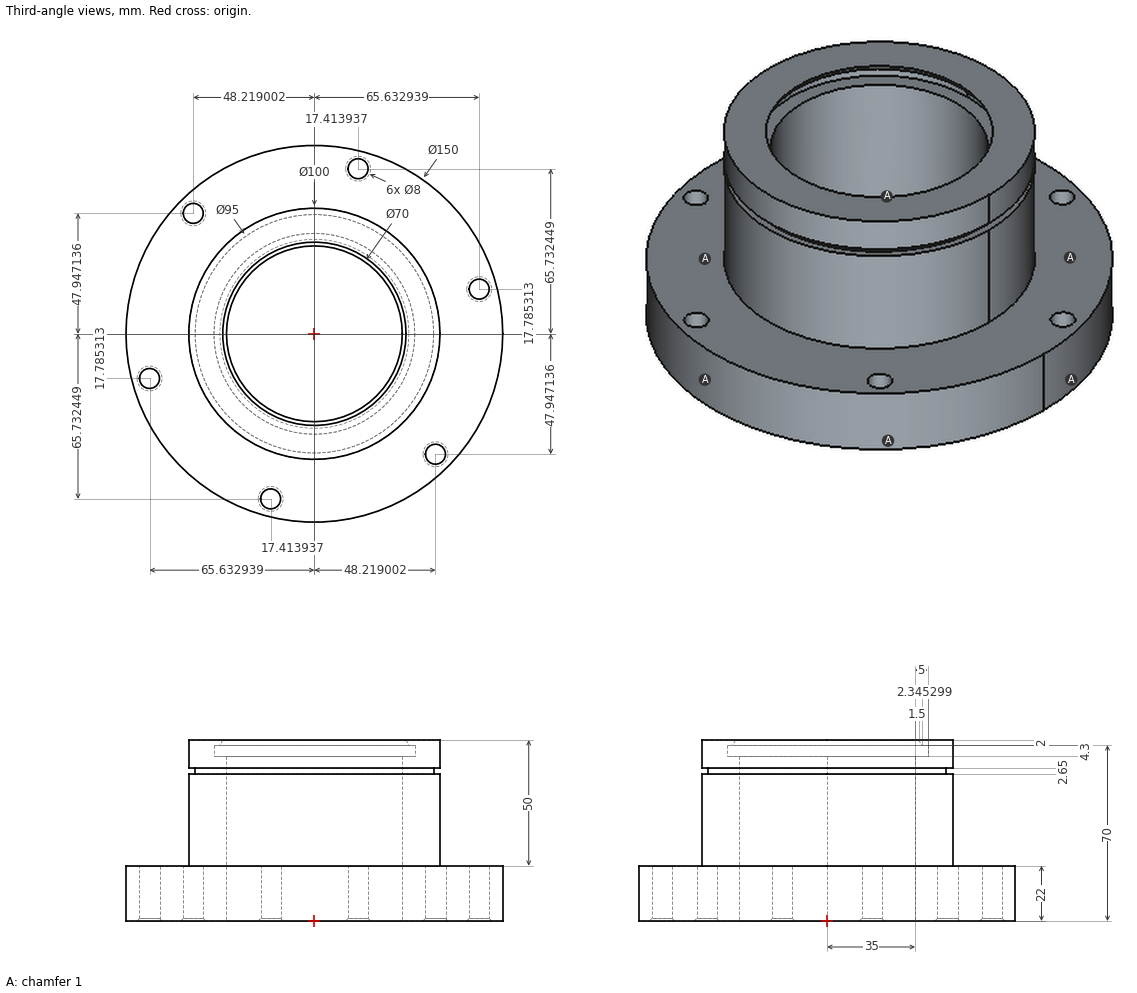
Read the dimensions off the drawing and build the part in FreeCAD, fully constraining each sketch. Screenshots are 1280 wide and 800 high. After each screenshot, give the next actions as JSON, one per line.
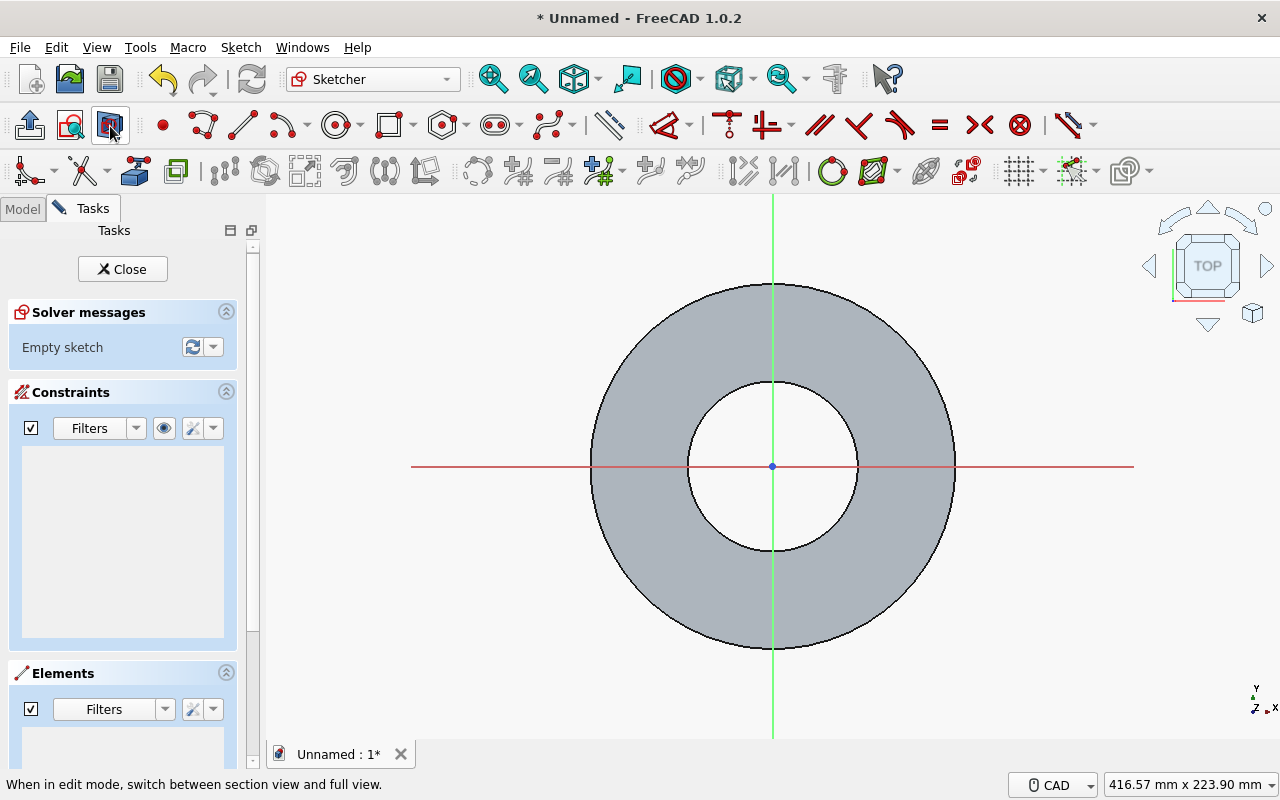
{"action": "left_click", "coordinate": [336, 126]}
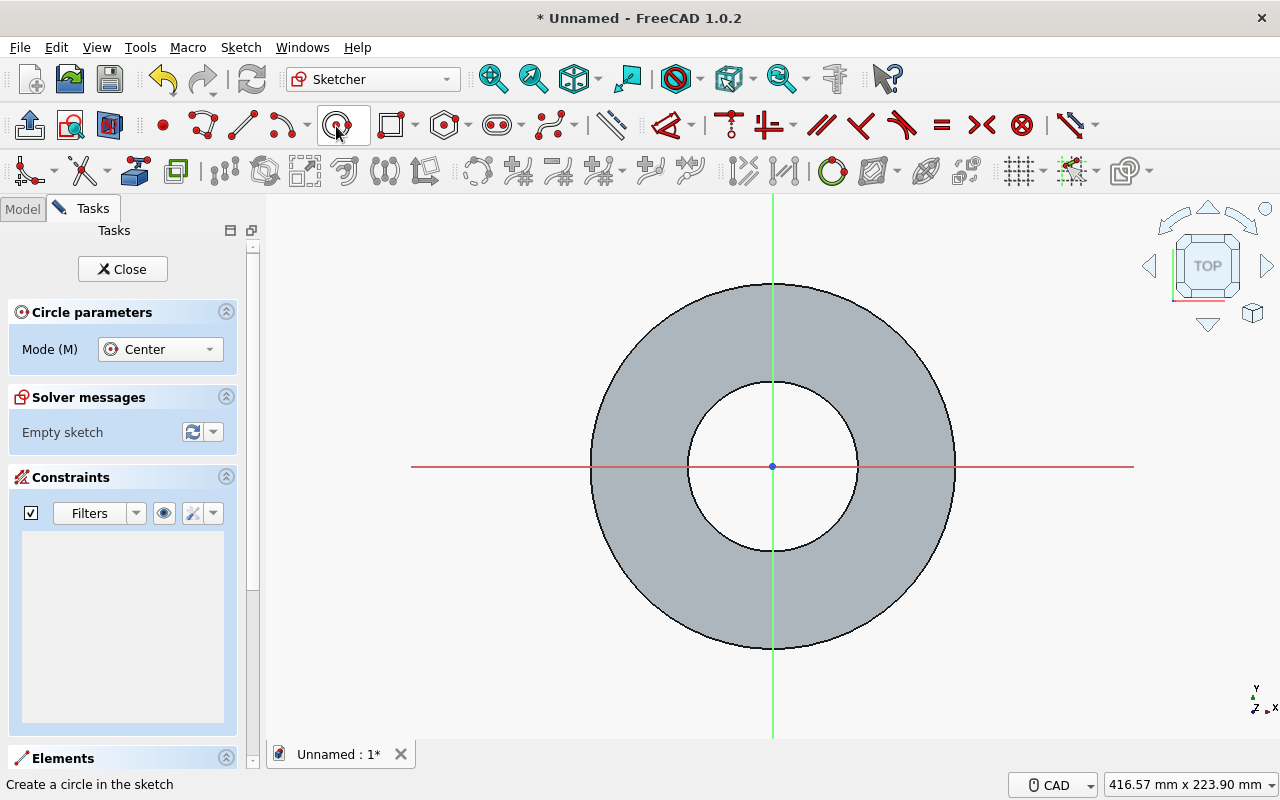
{"action": "scroll", "coordinate": [815, 306], "scroll_direction": "up", "scroll_amount": 5}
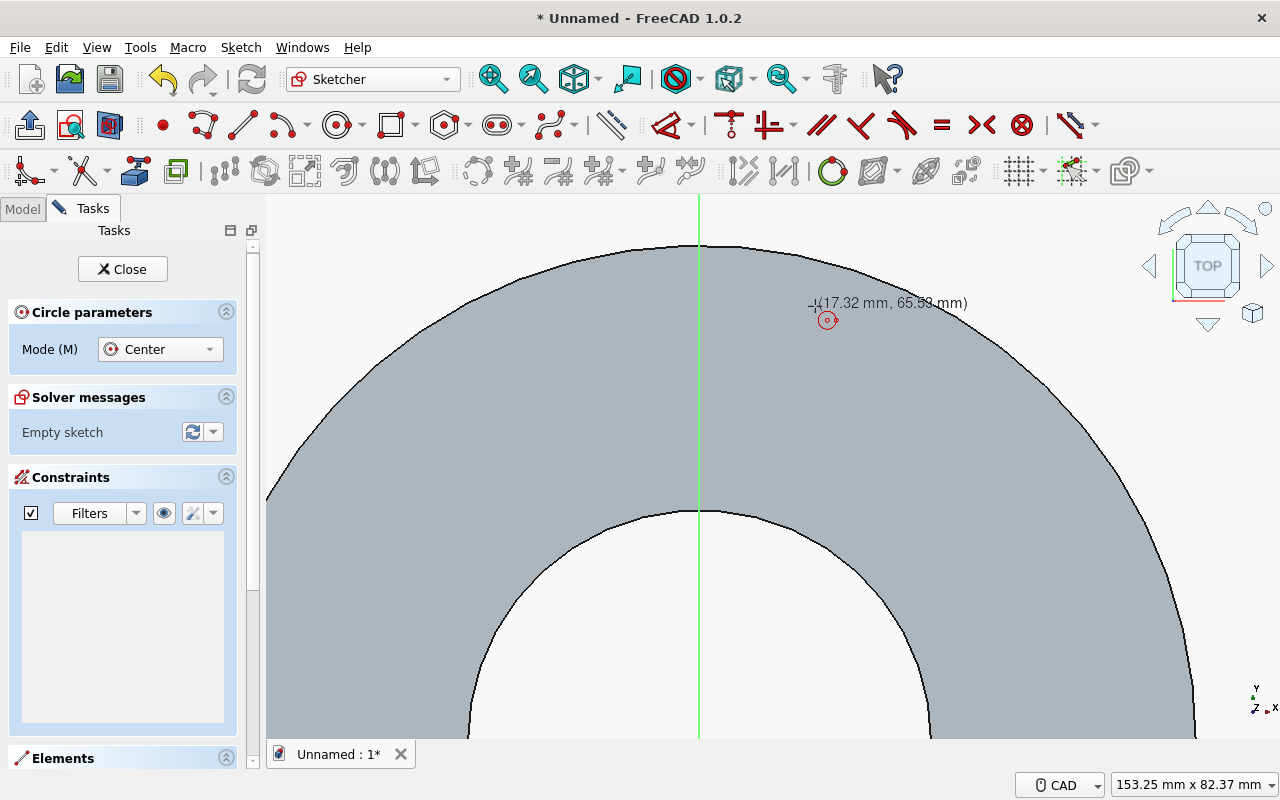
{"action": "left_click", "coordinate": [815, 307]}
{"action": "left_click", "coordinate": [833, 288]}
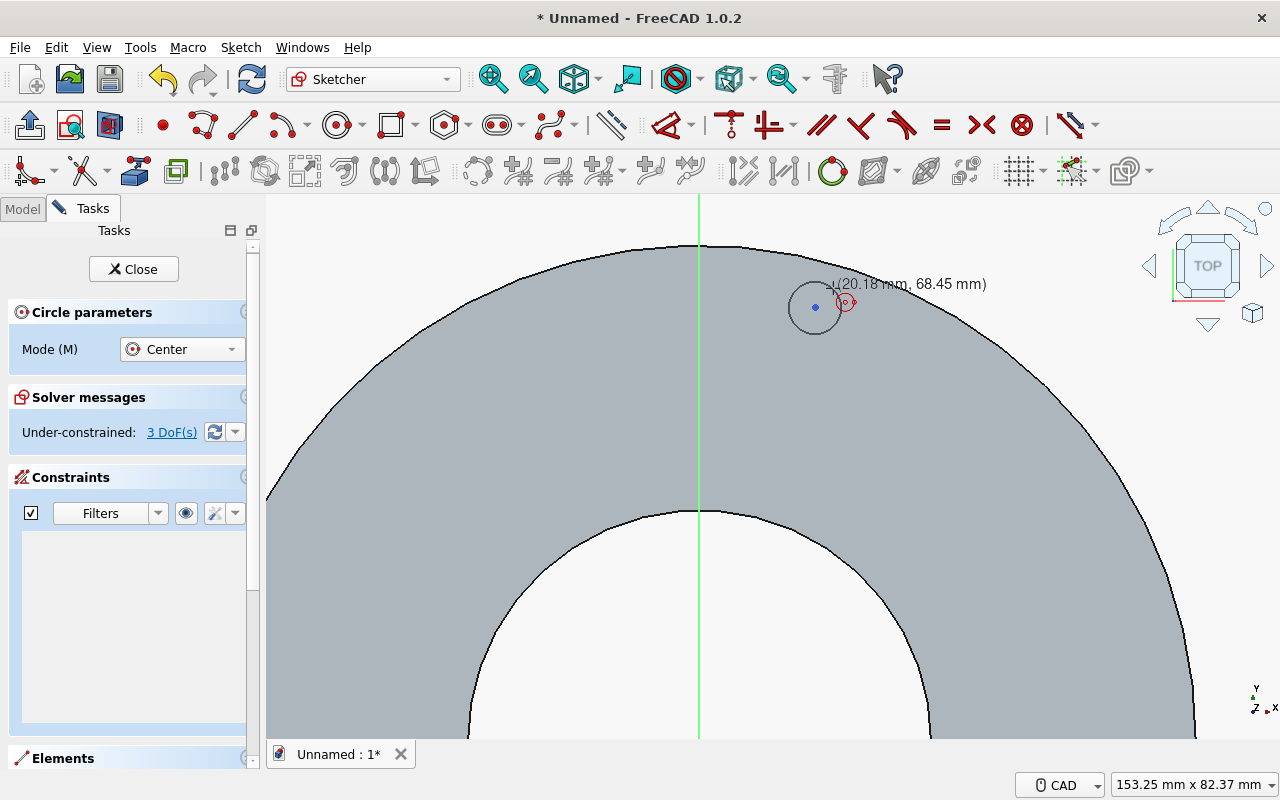
{"action": "left_click", "coordinate": [380, 425]}
{"action": "left_click", "coordinate": [399, 406]}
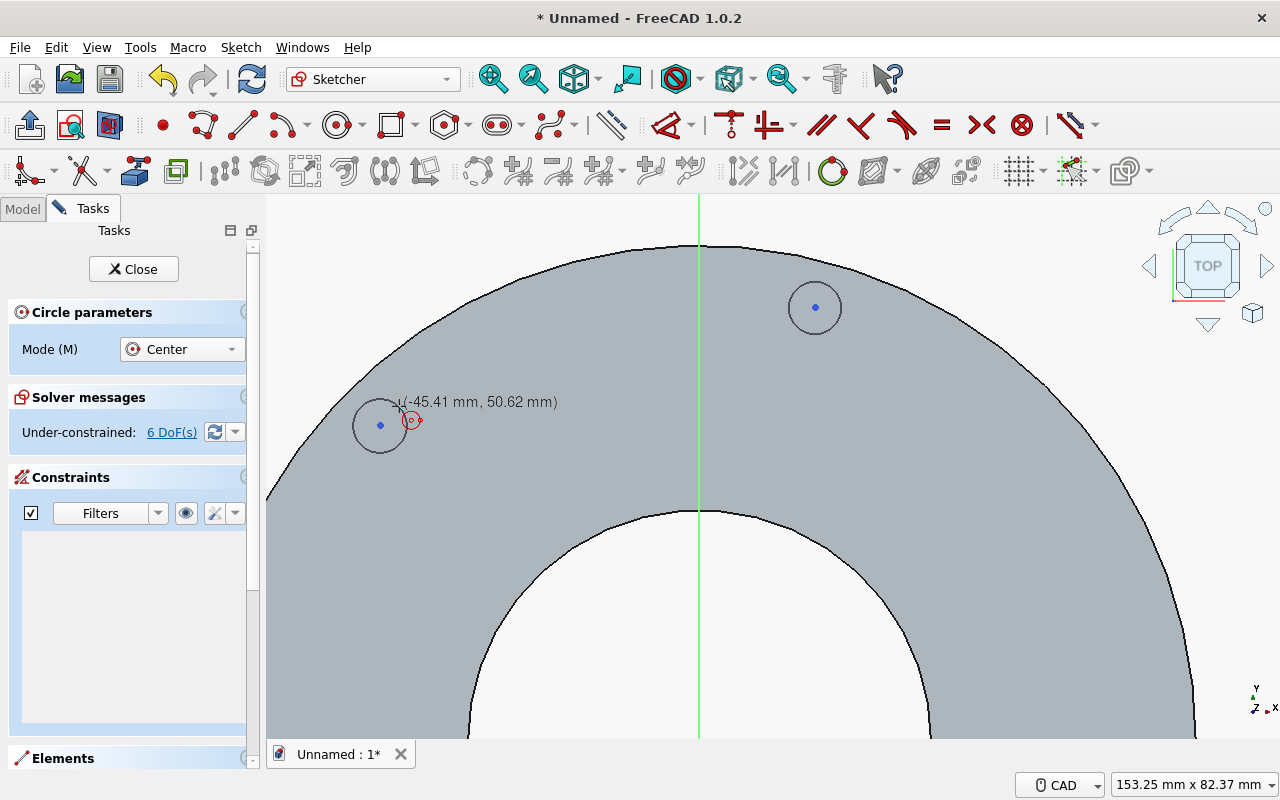
{"action": "scroll", "coordinate": [707, 306], "scroll_direction": "down", "scroll_amount": 5}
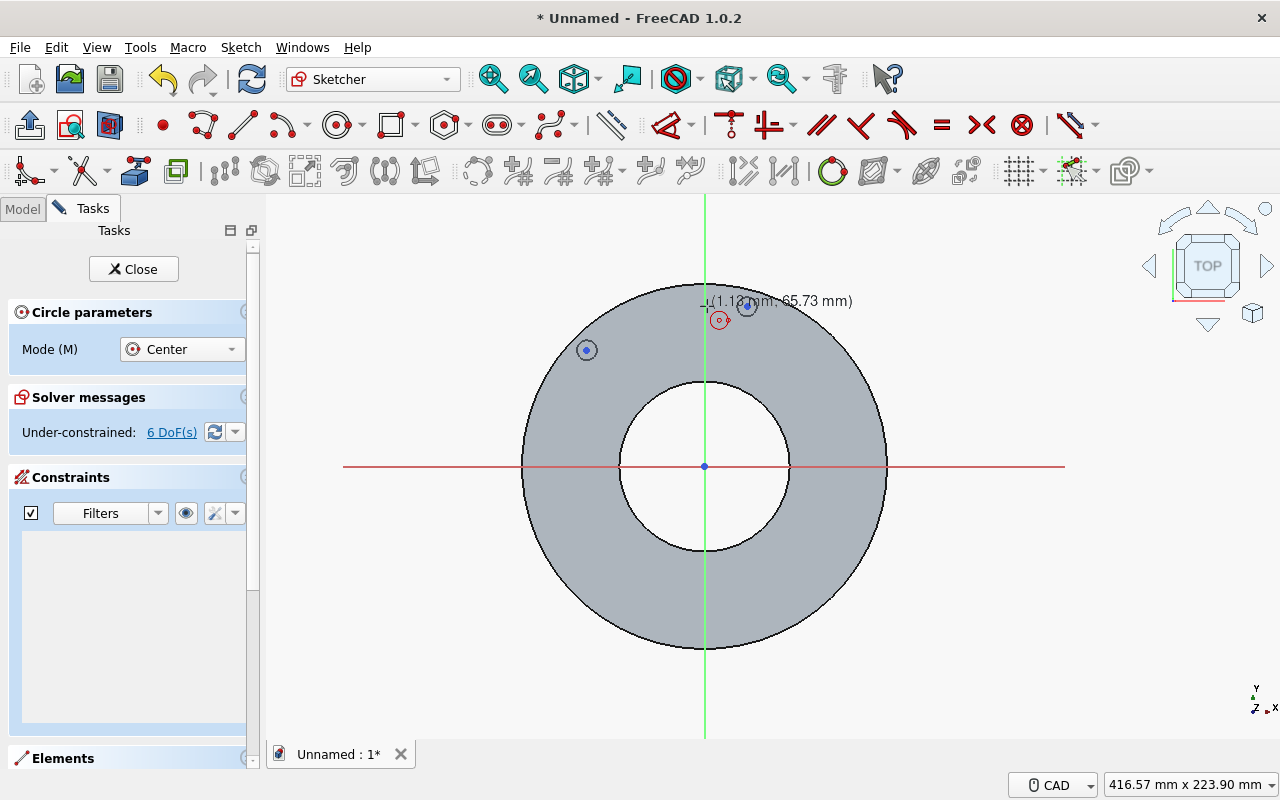
{"action": "scroll", "coordinate": [545, 510], "scroll_direction": "up", "scroll_amount": 5}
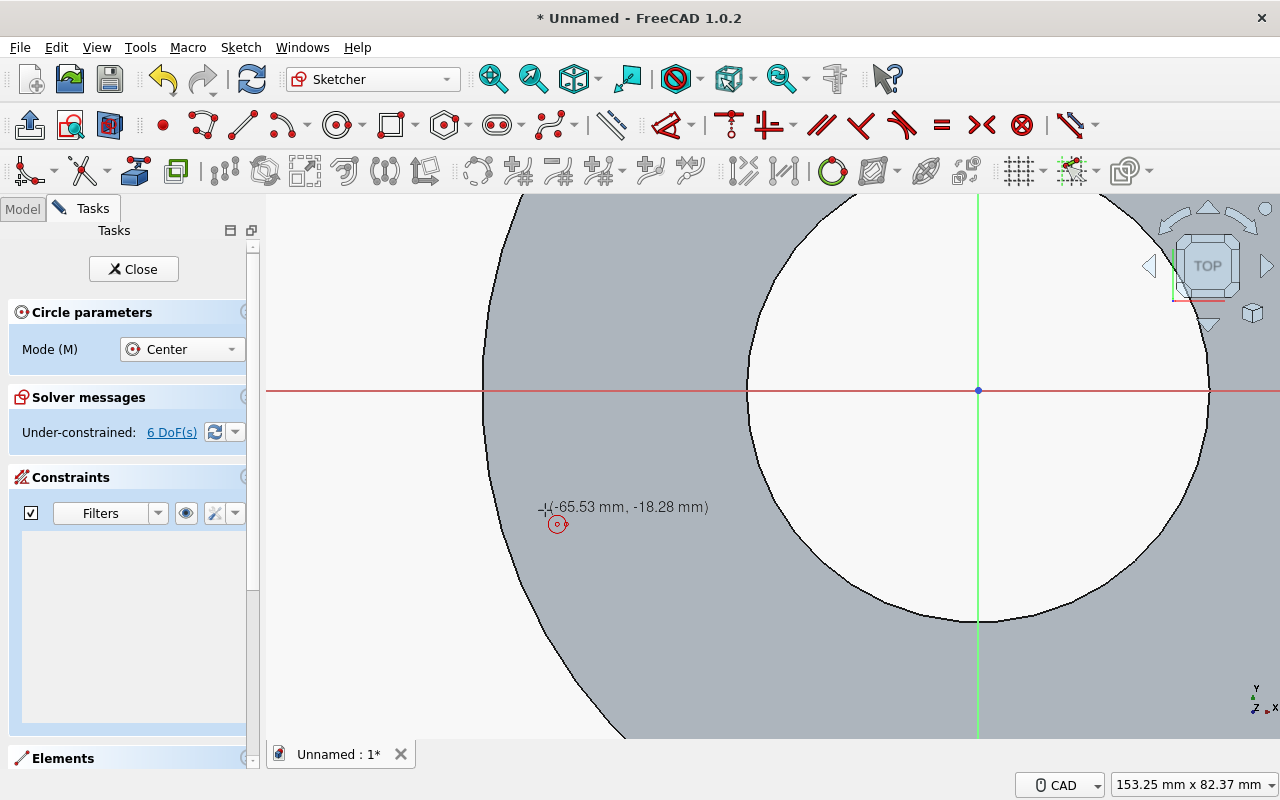
{"action": "left_click", "coordinate": [544, 508]}
{"action": "left_click", "coordinate": [563, 490]}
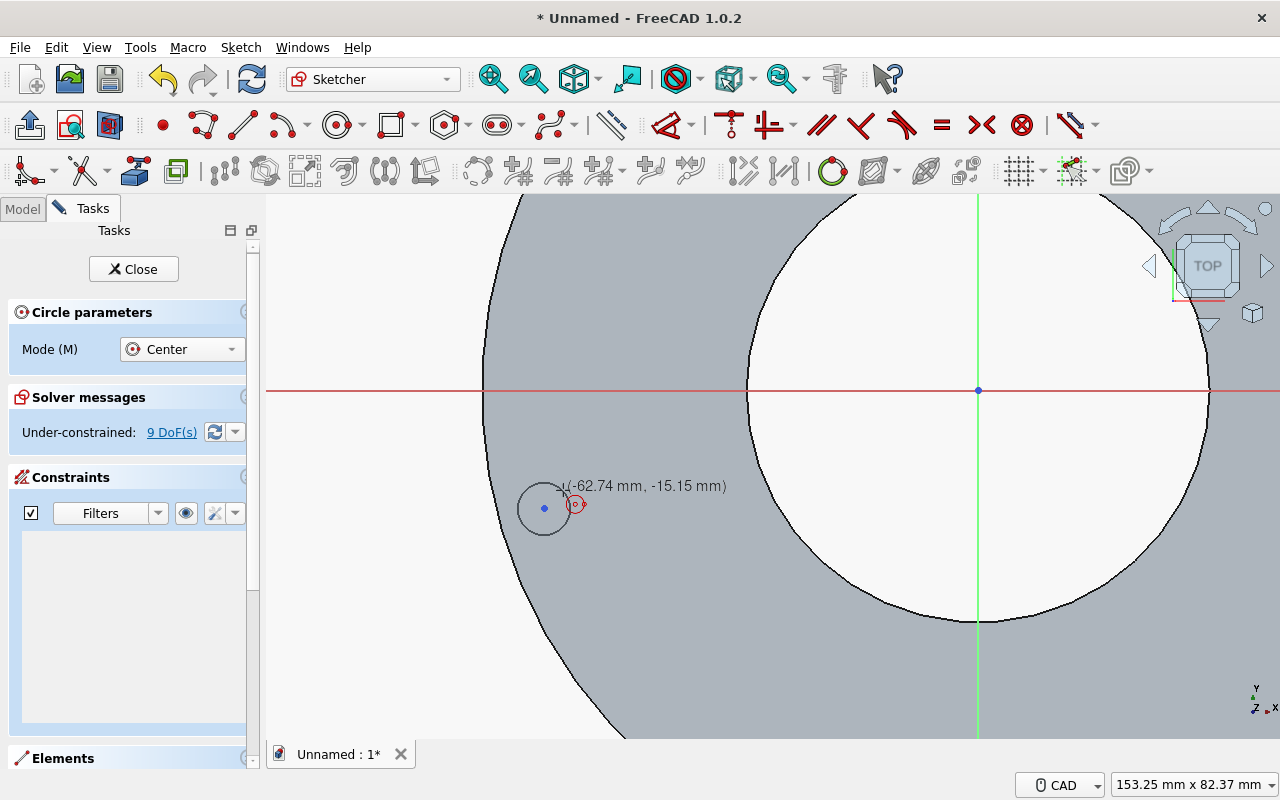
{"action": "scroll", "coordinate": [545, 511], "scroll_direction": "down", "scroll_amount": 5}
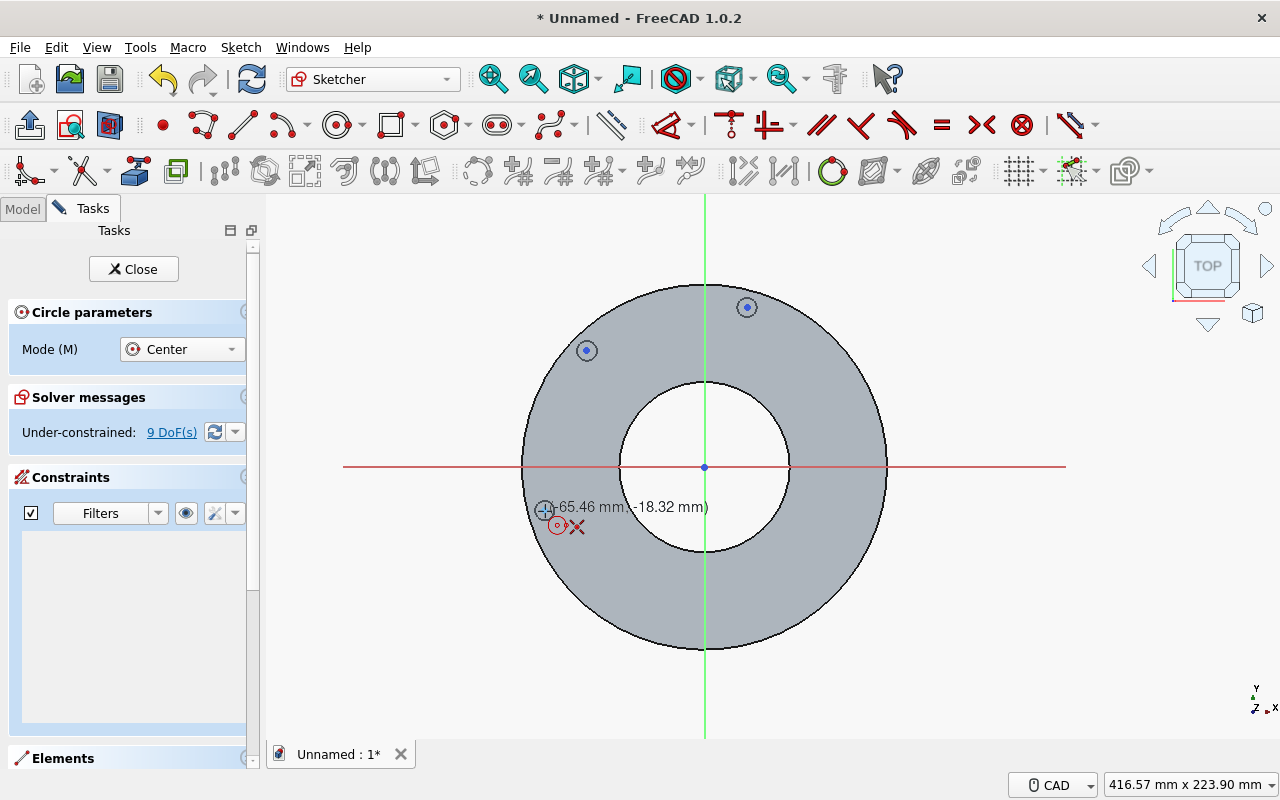
{"action": "scroll", "coordinate": [662, 627], "scroll_direction": "up", "scroll_amount": 5}